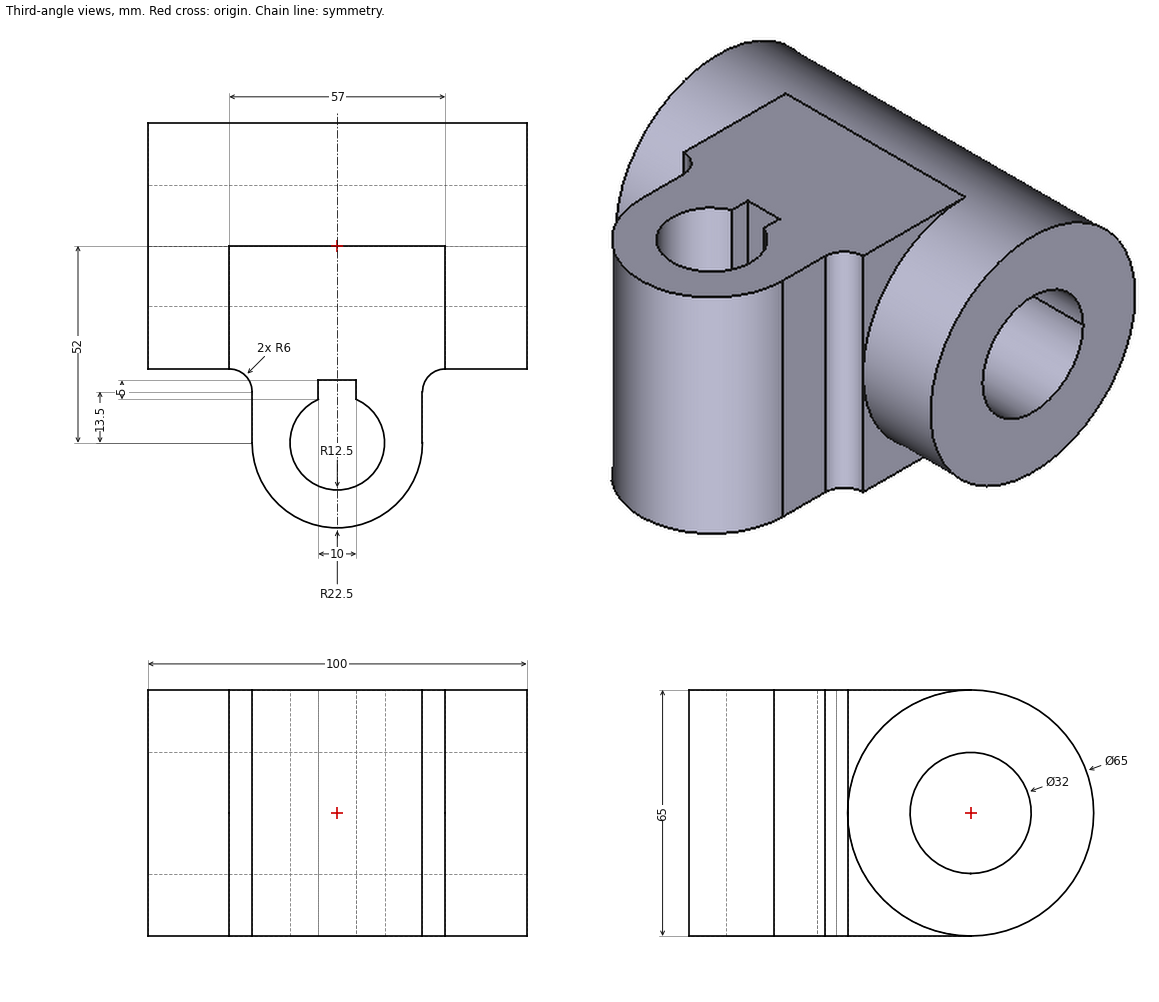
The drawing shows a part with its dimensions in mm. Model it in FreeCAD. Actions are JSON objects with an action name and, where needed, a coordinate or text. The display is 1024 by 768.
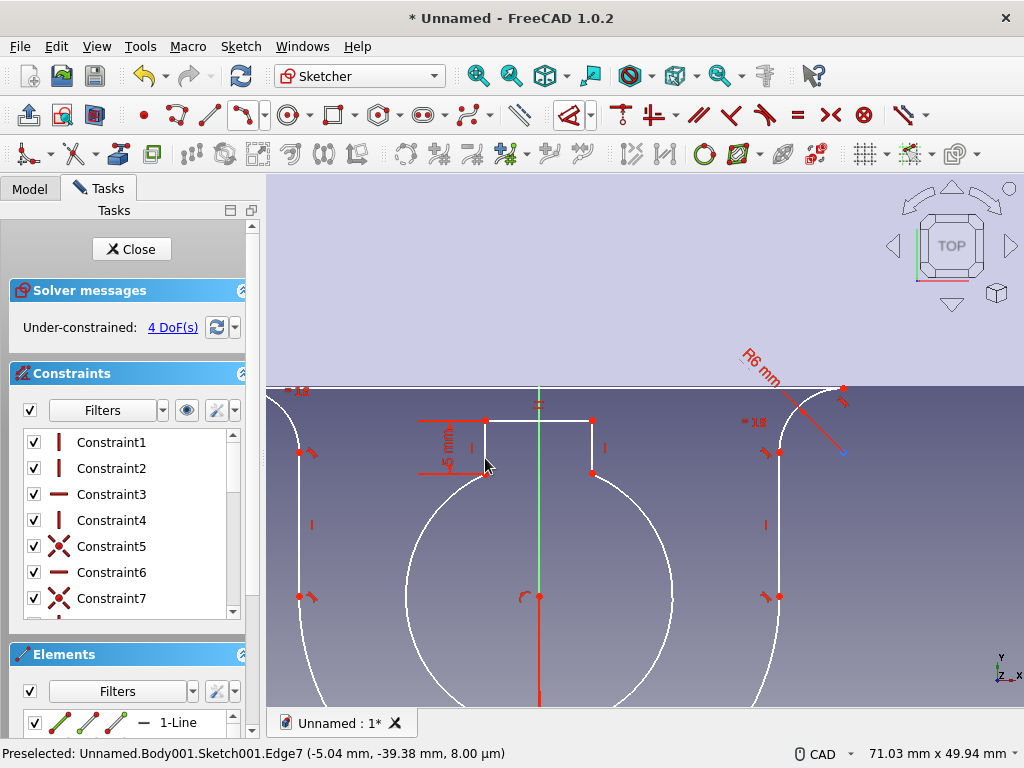
{"action": "left_click", "coordinate": [592, 437]}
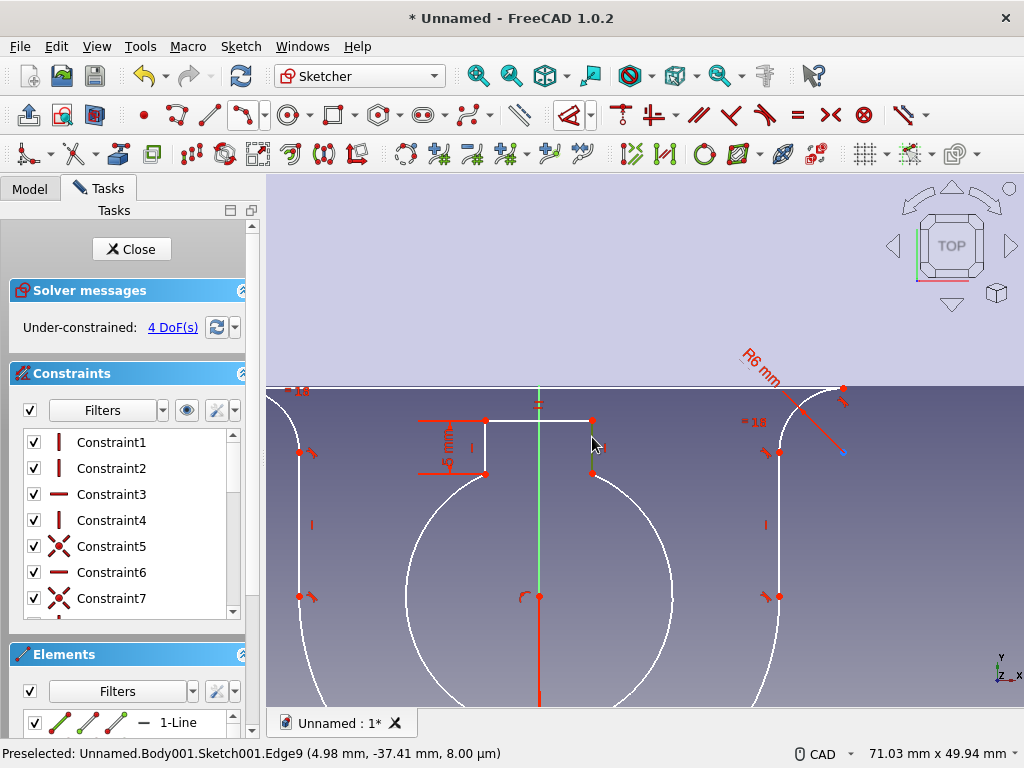
{"action": "key", "text": "i"}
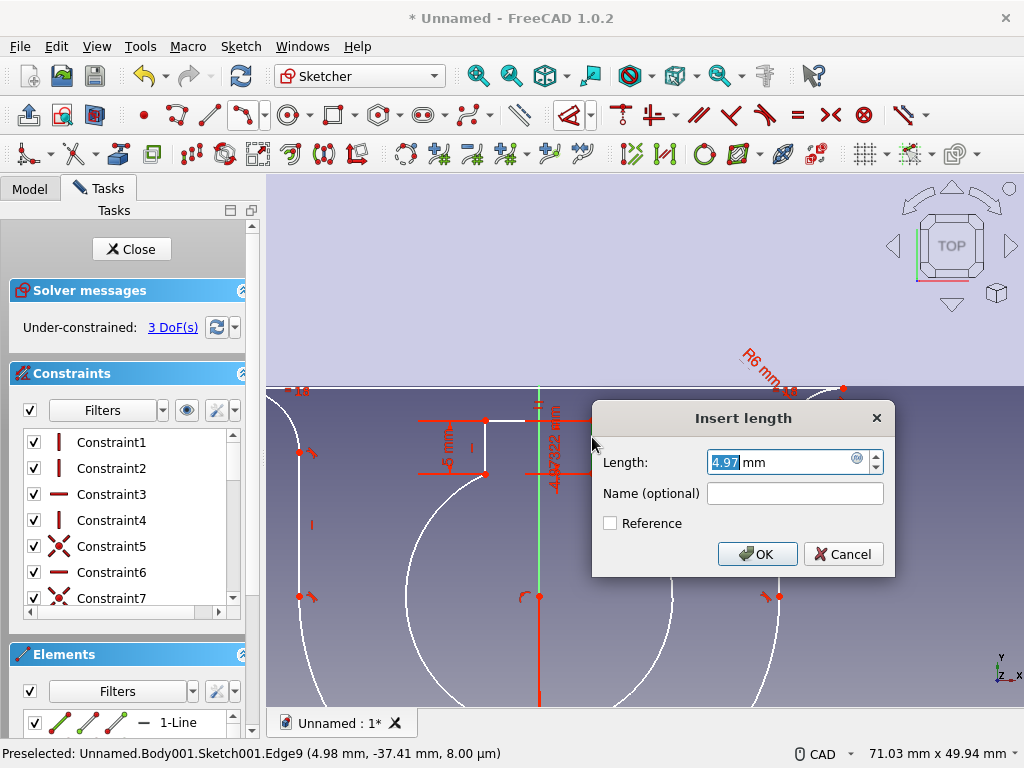
{"action": "type", "text": "5"}
{"action": "key", "text": "Return"}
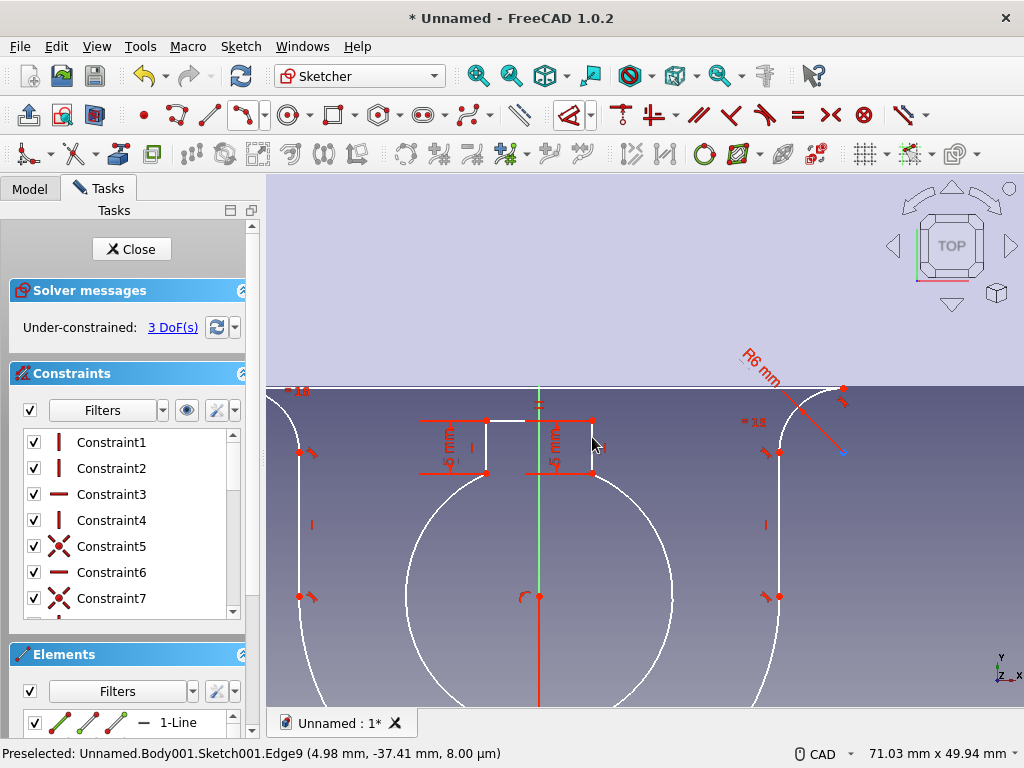
{"action": "left_click", "coordinate": [518, 421]}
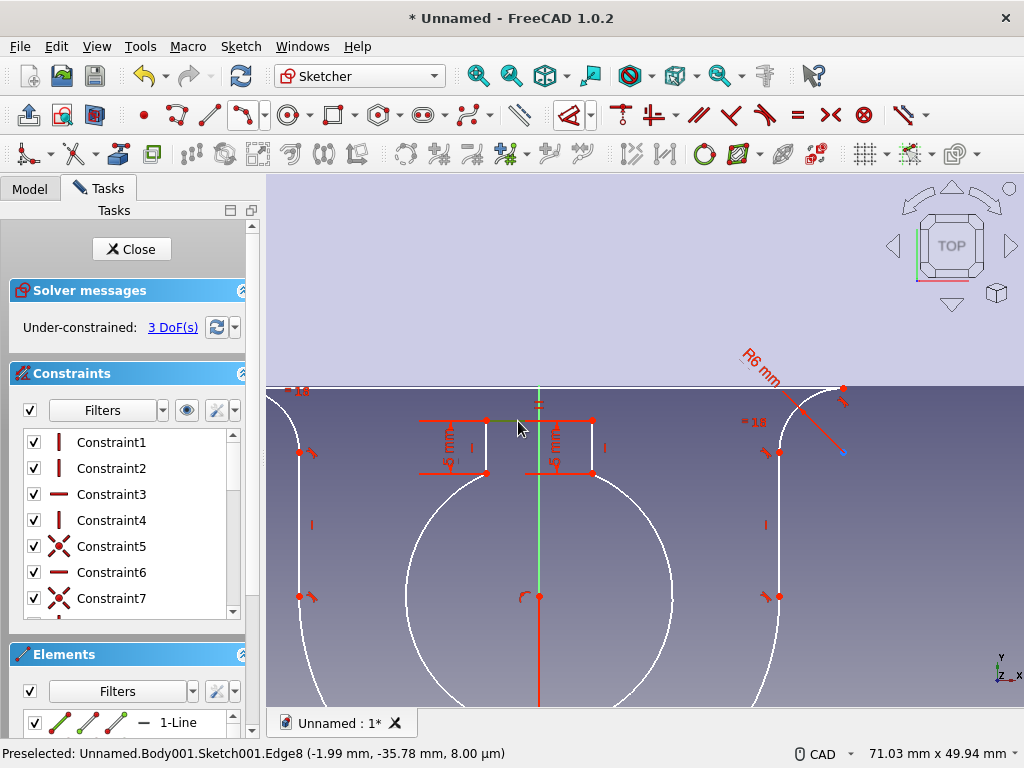
{"action": "key", "text": "l"}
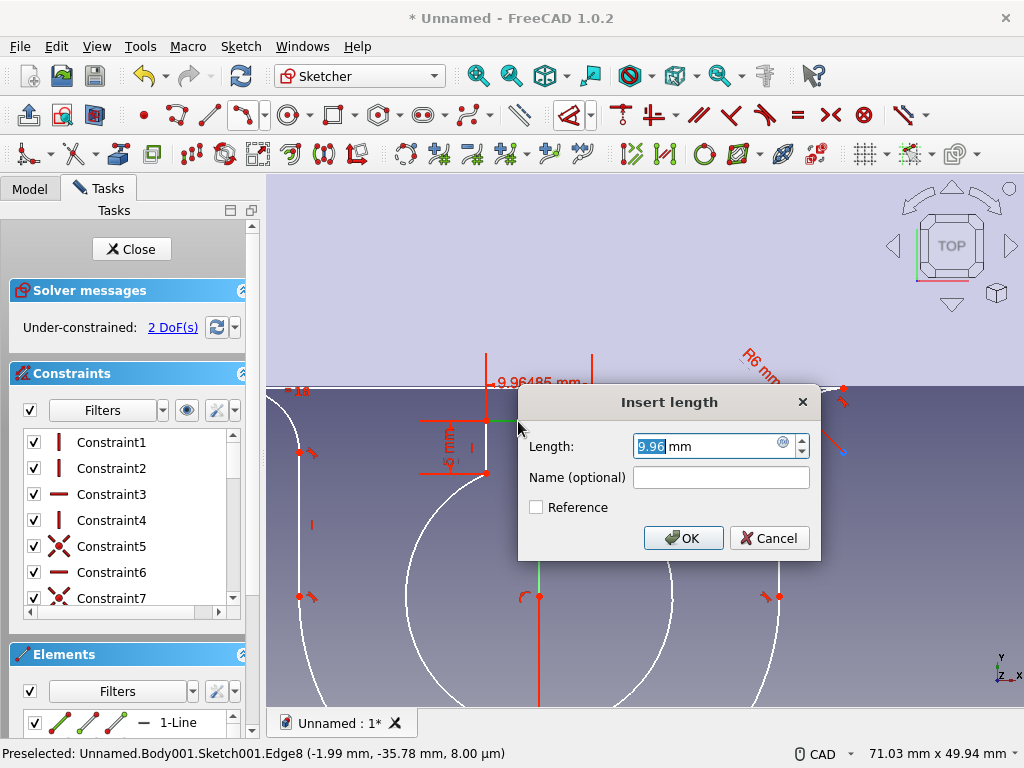
{"action": "type", "text": "10"}
{"action": "key", "text": "Return"}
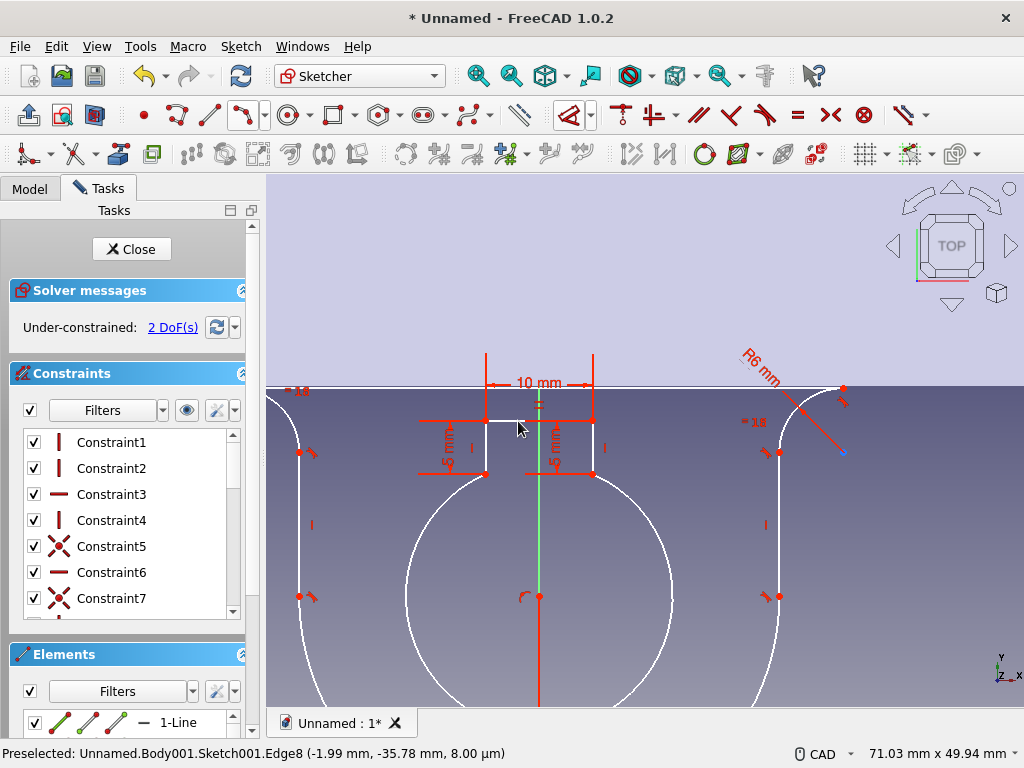
{"action": "left_click", "coordinate": [299, 596]}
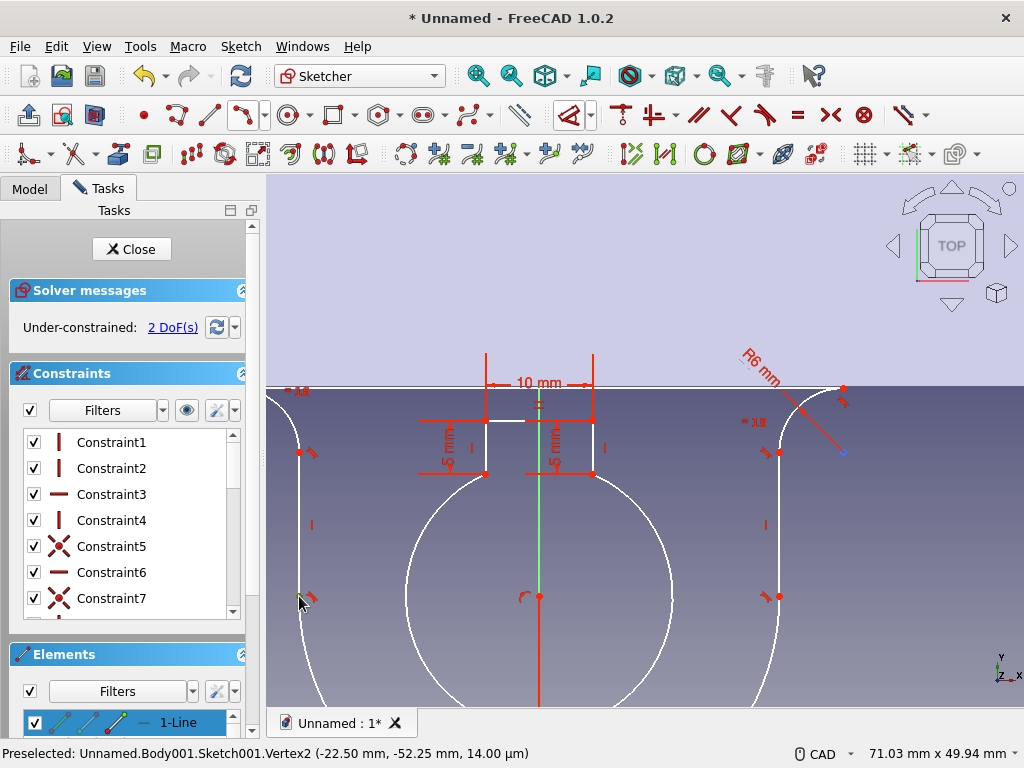
{"action": "left_click", "coordinate": [590, 116]}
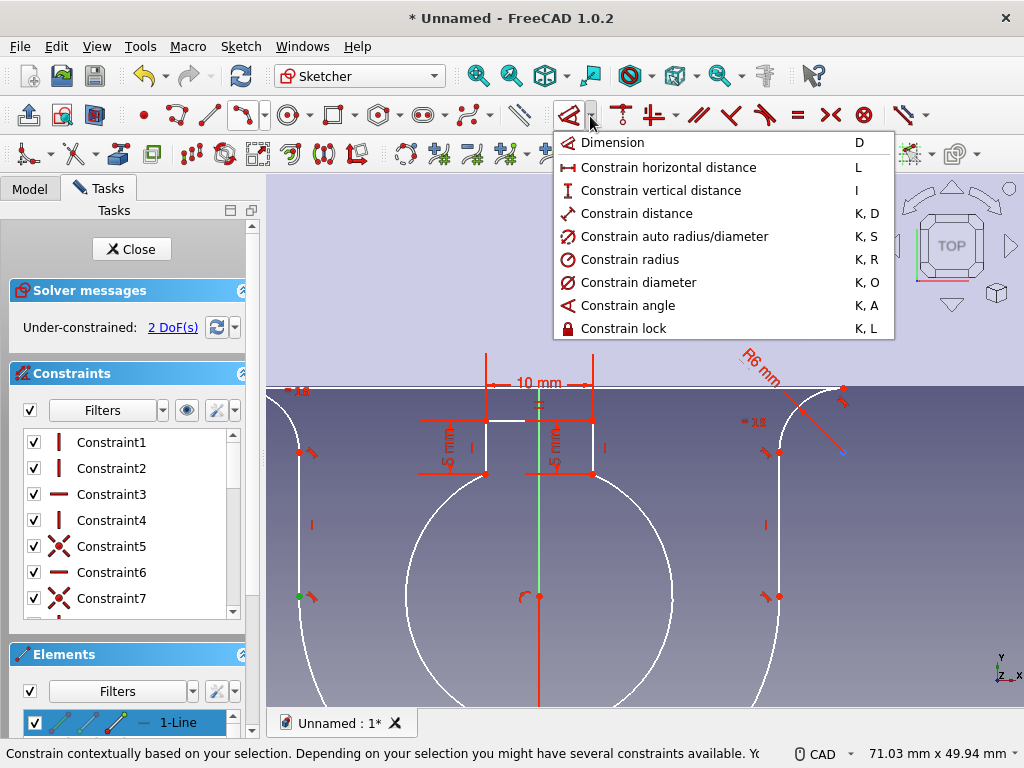
{"action": "left_click", "coordinate": [724, 190]}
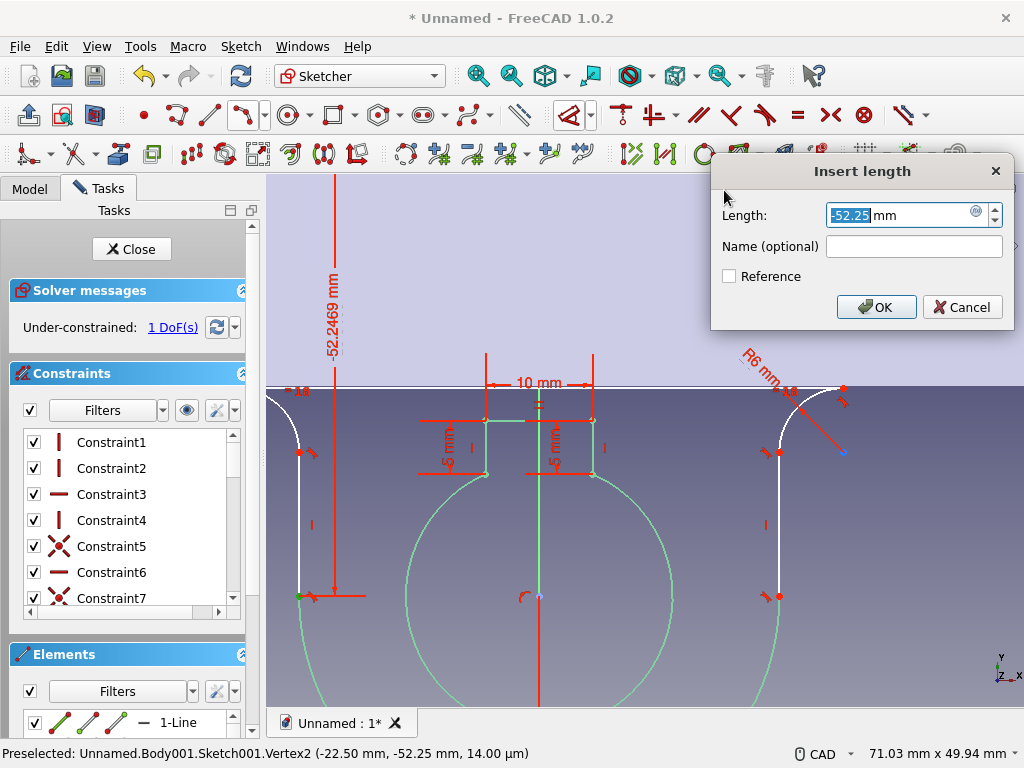
{"action": "type", "text": "-52"}
{"action": "key", "text": "Return"}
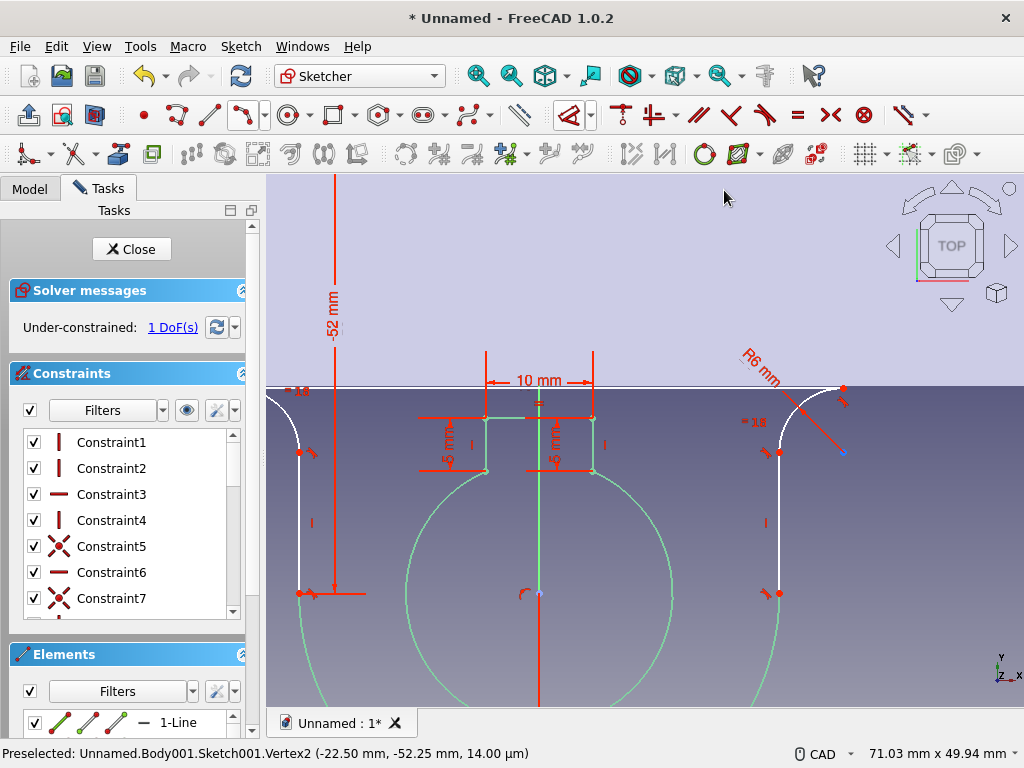
{"action": "left_click", "coordinate": [299, 495]}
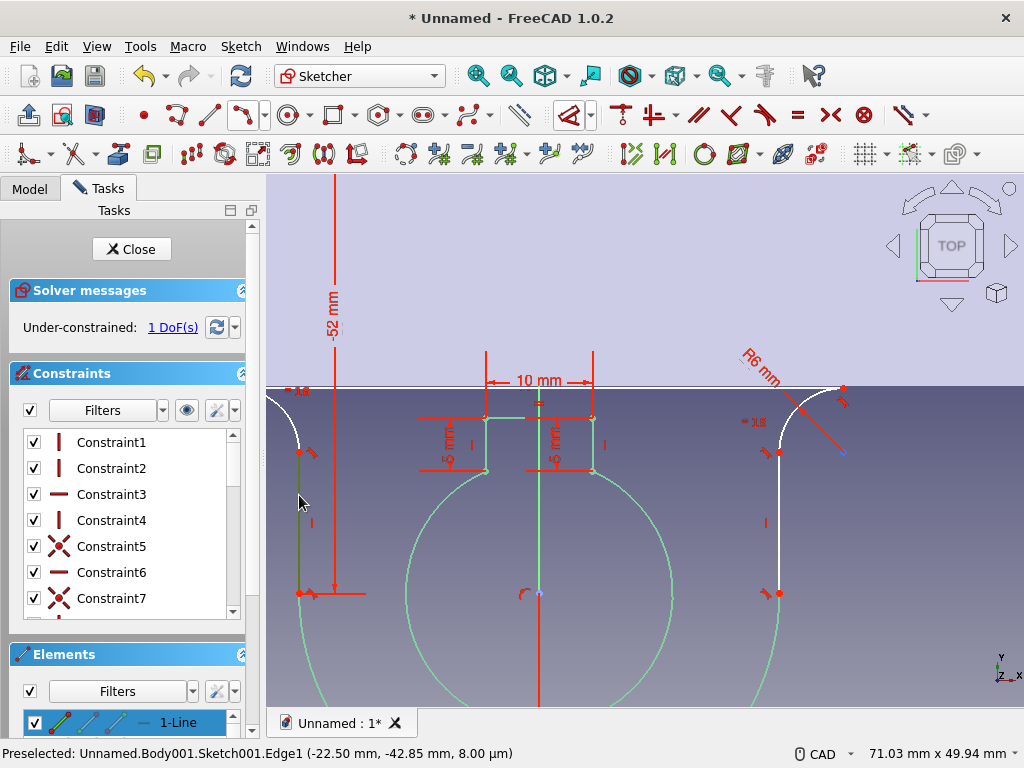
{"action": "key", "text": "i"}